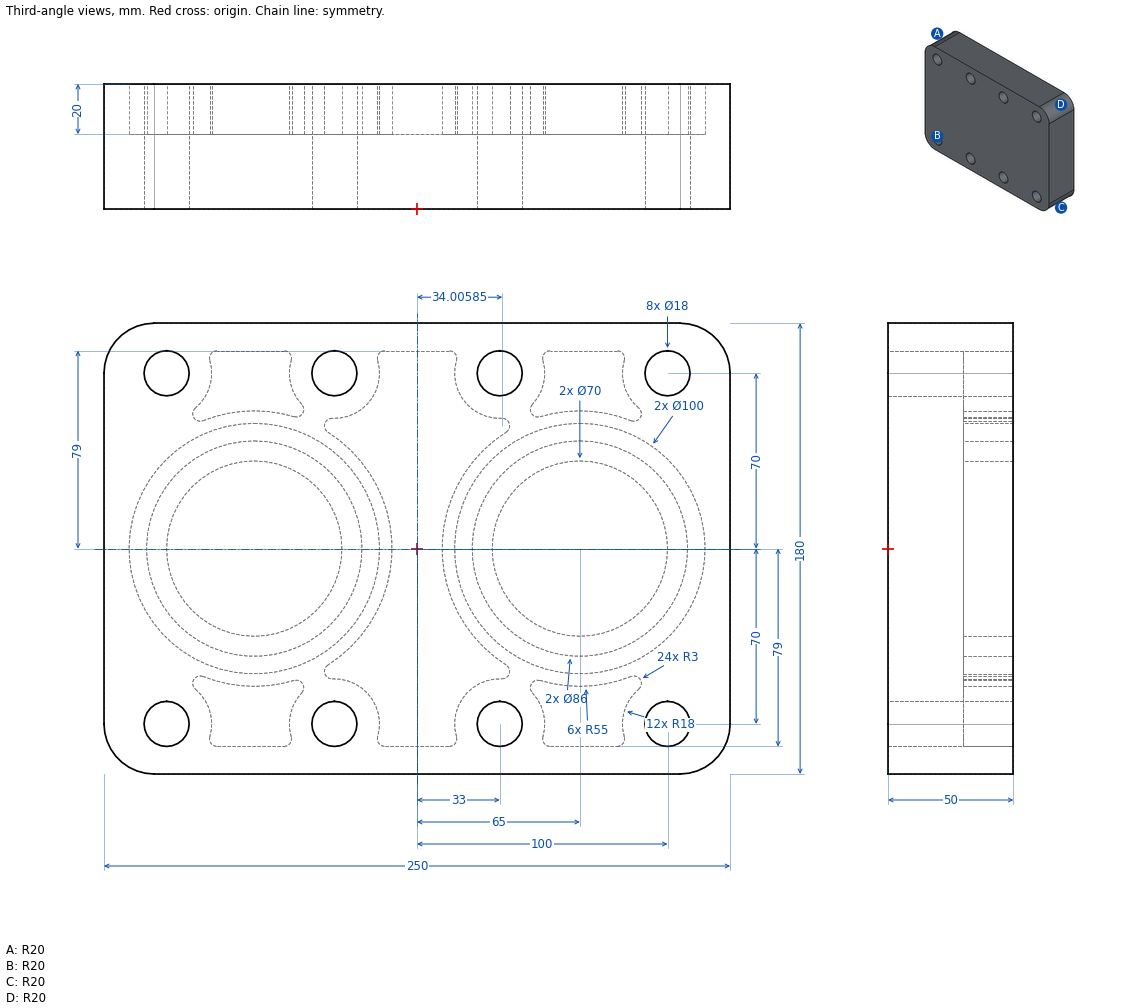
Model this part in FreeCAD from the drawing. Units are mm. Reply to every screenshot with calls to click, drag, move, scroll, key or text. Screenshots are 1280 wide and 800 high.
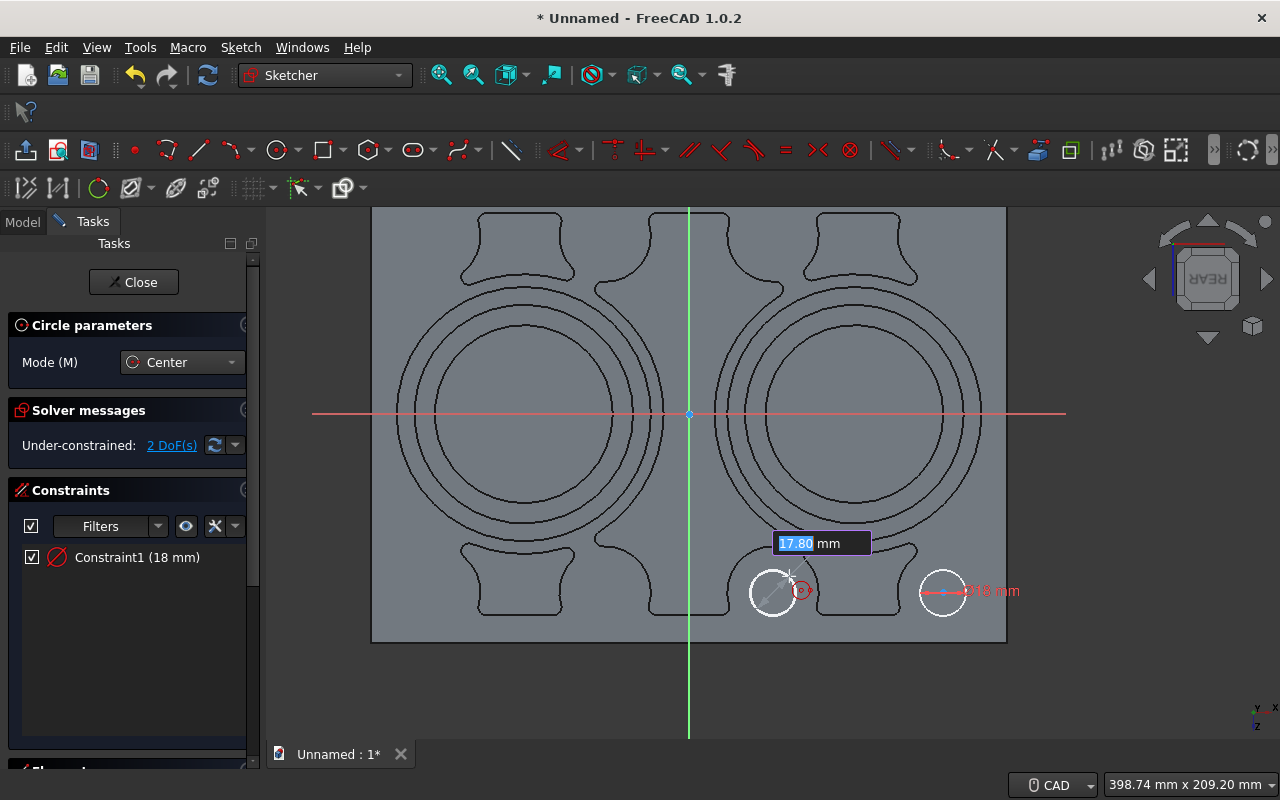
text(18)
key(Return)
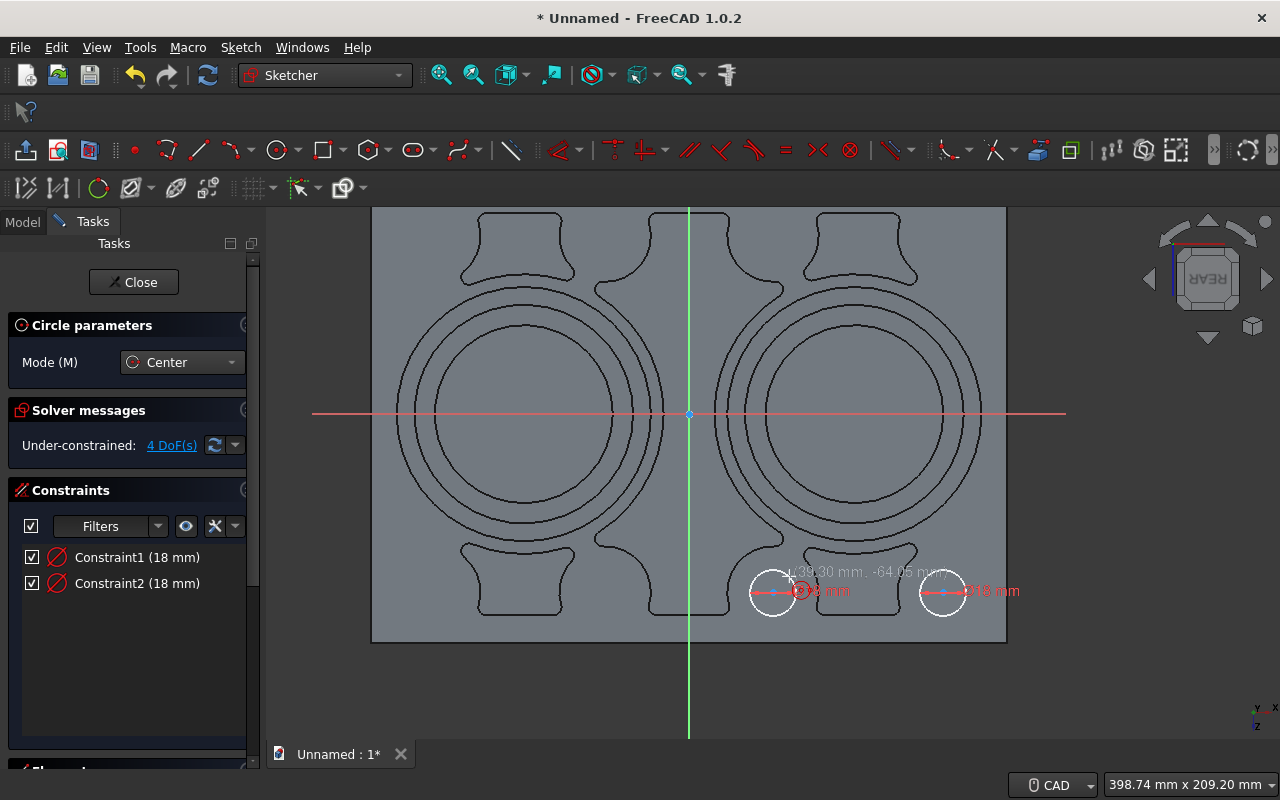
click(605, 592)
move(621, 576)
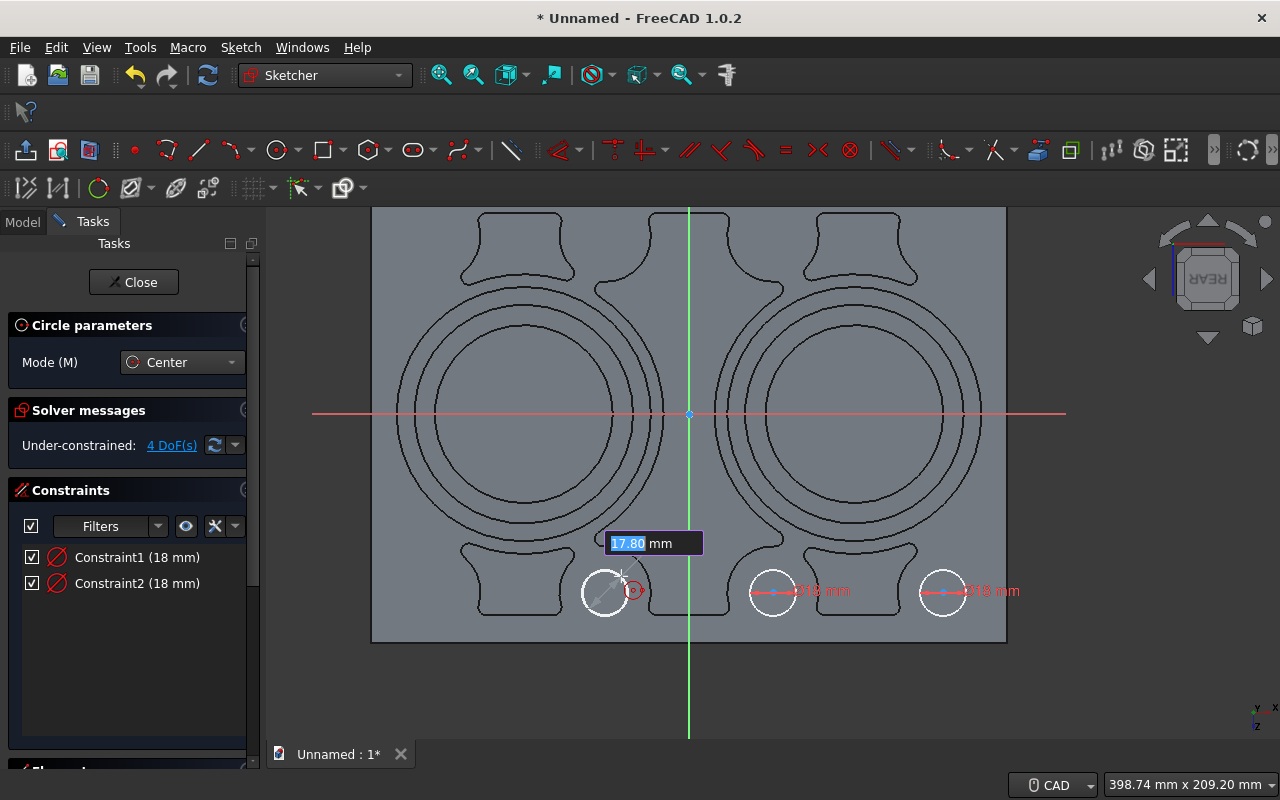
text(18)
key(Return)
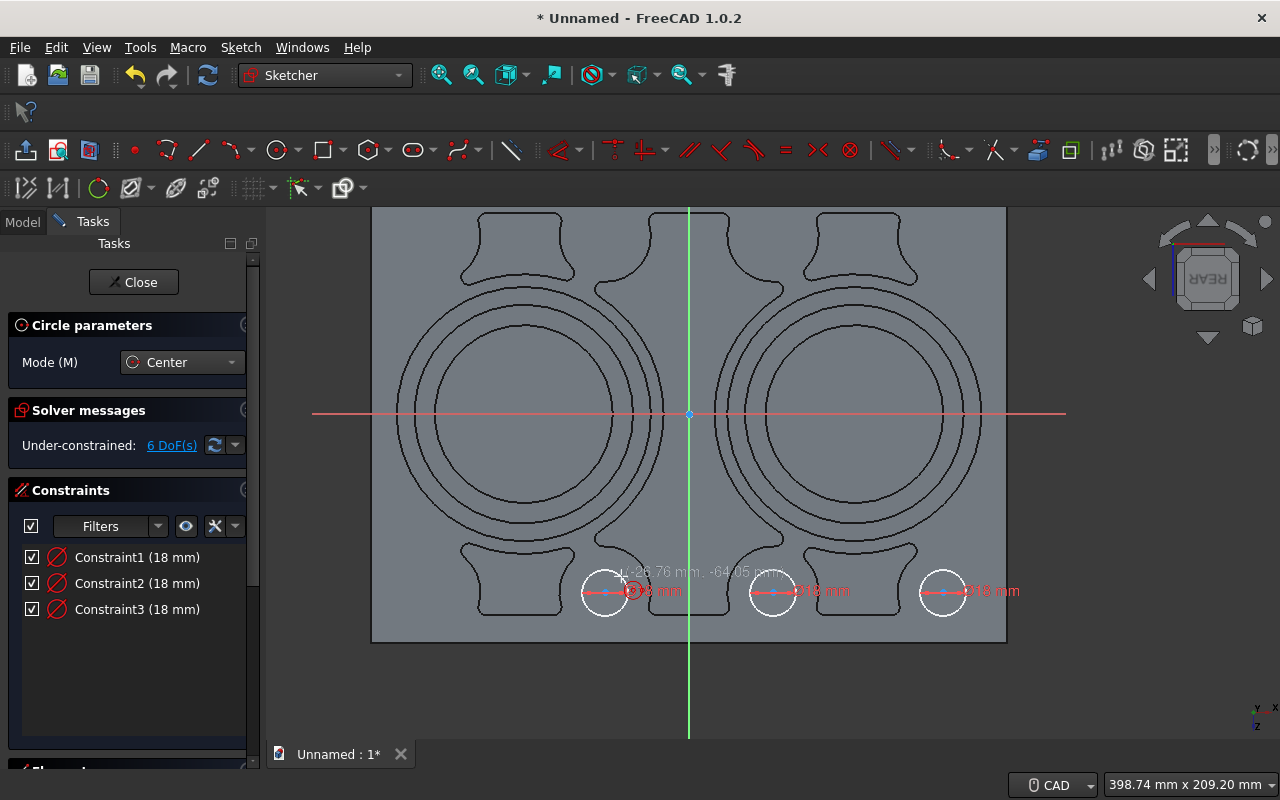
click(435, 592)
move(451, 576)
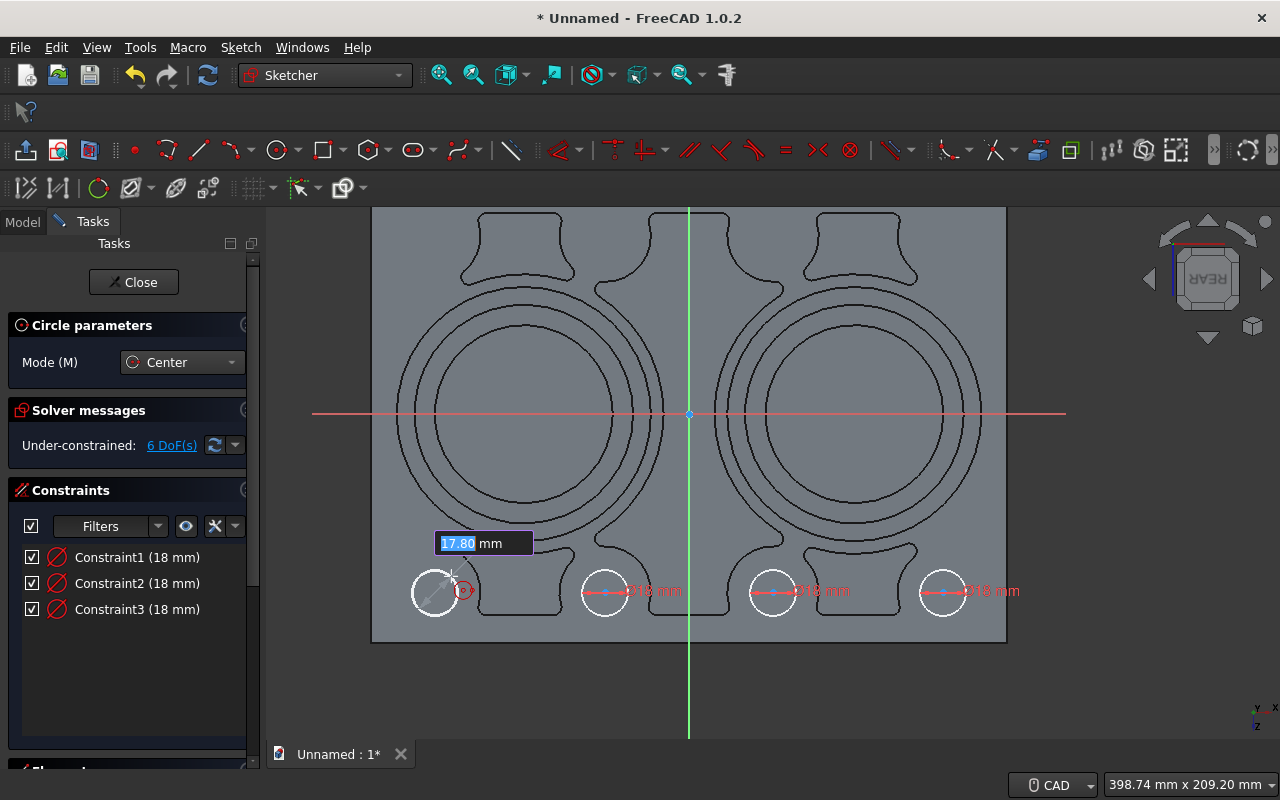
text(18)
key(Return)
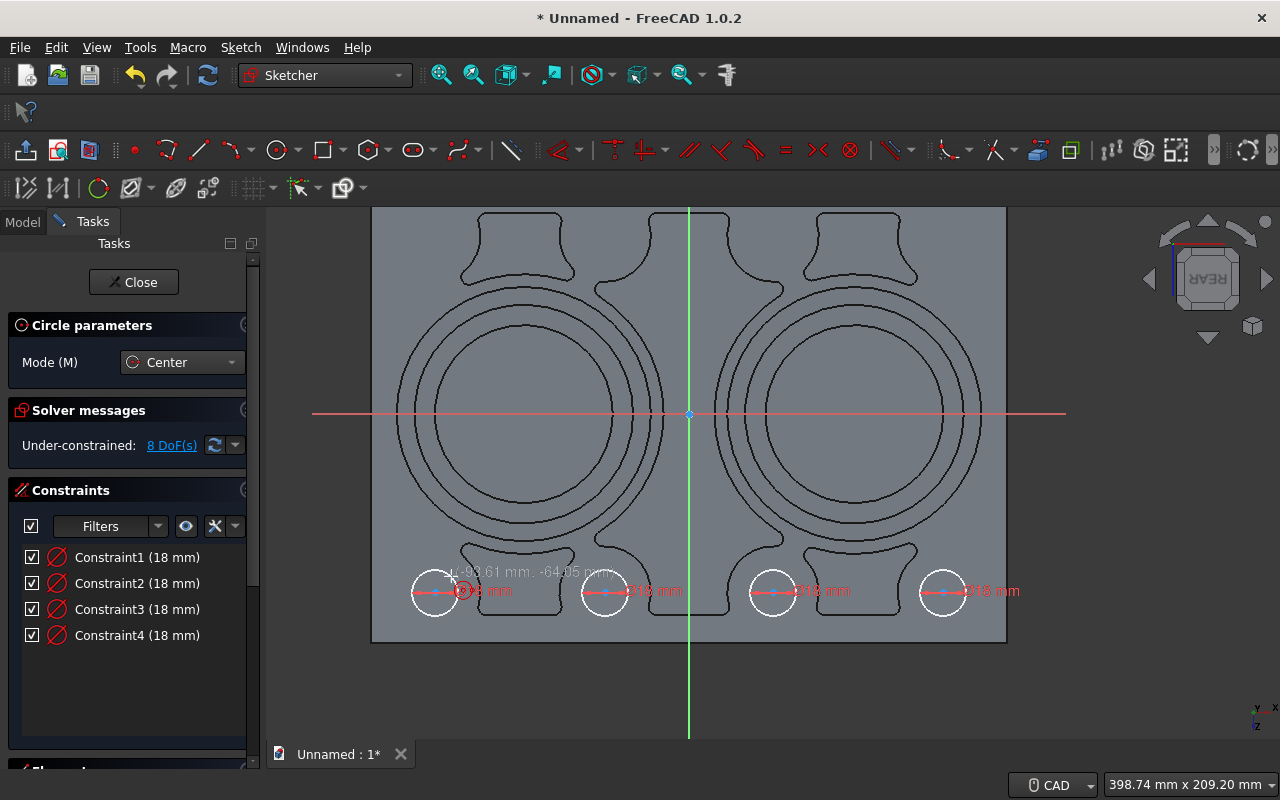
click(435, 236)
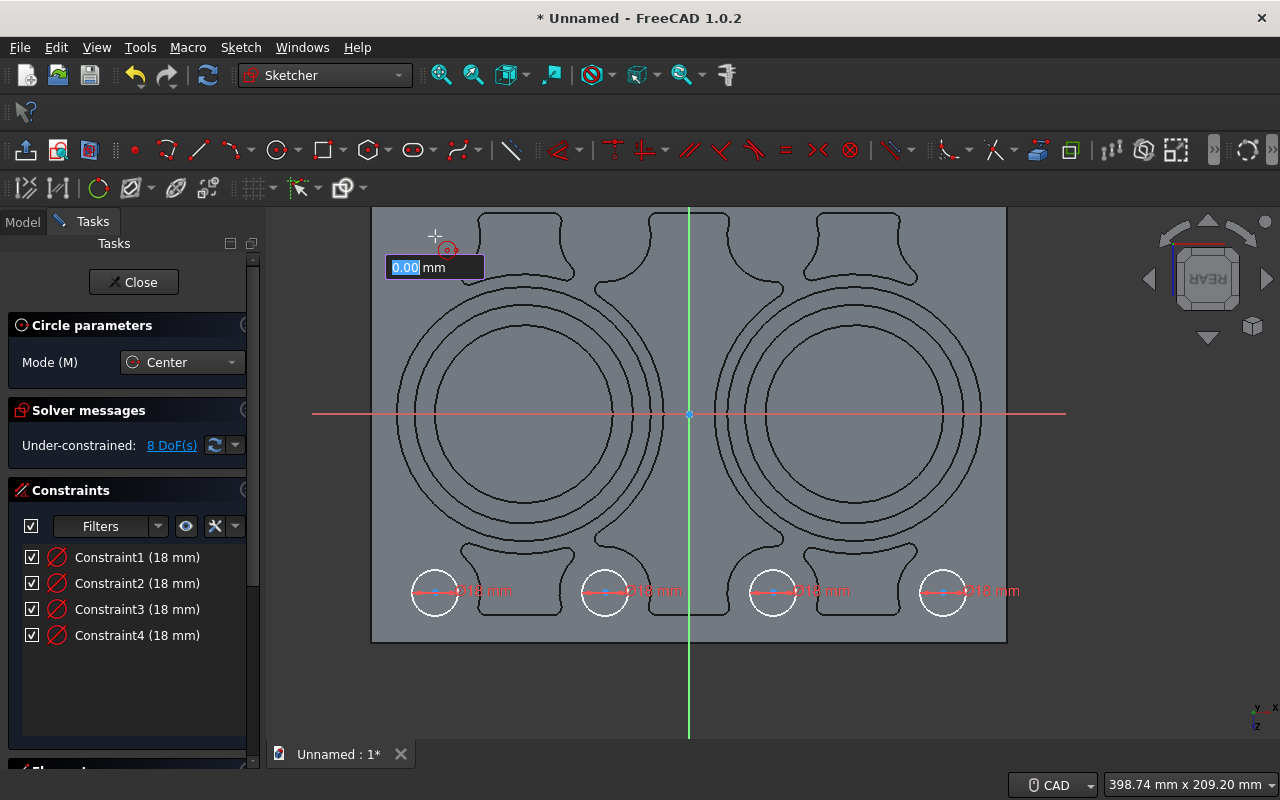
scroll(774, 711, down, 1)
move(510, 309)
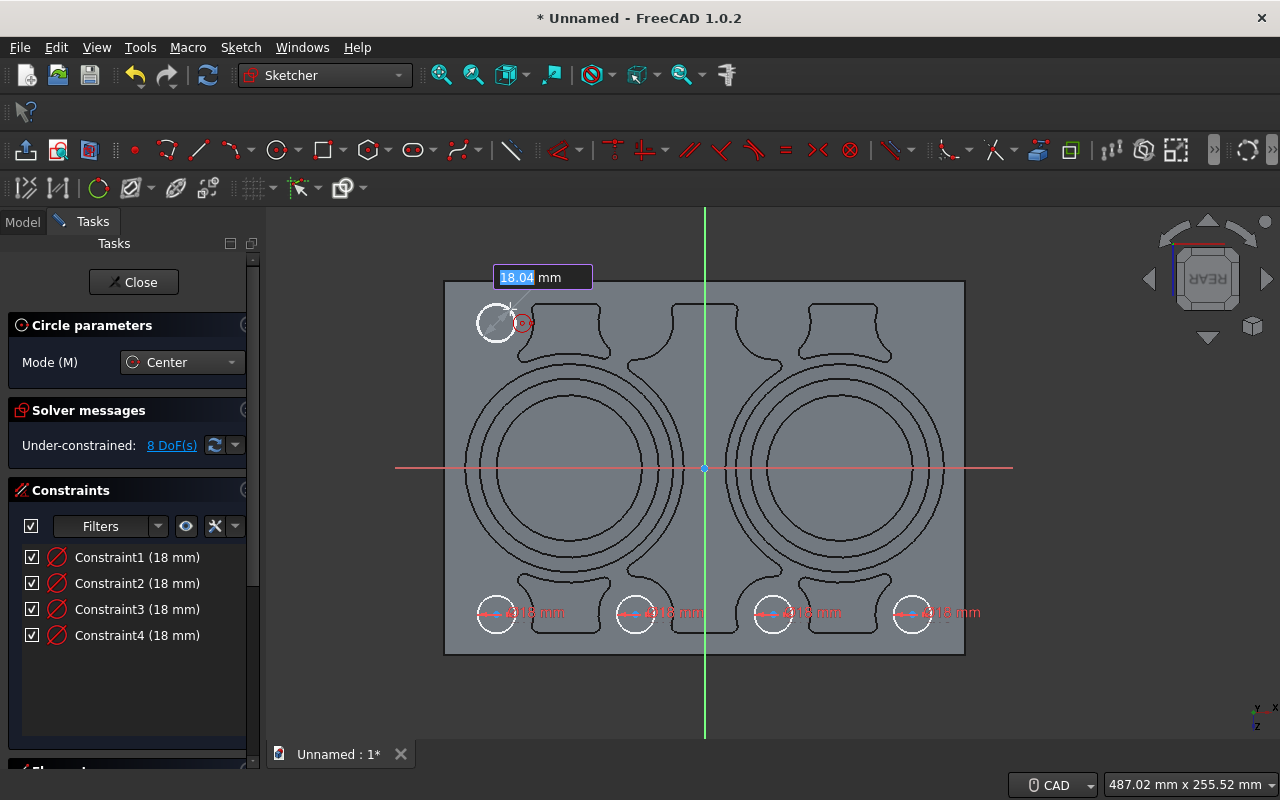
text(18)
key(Return)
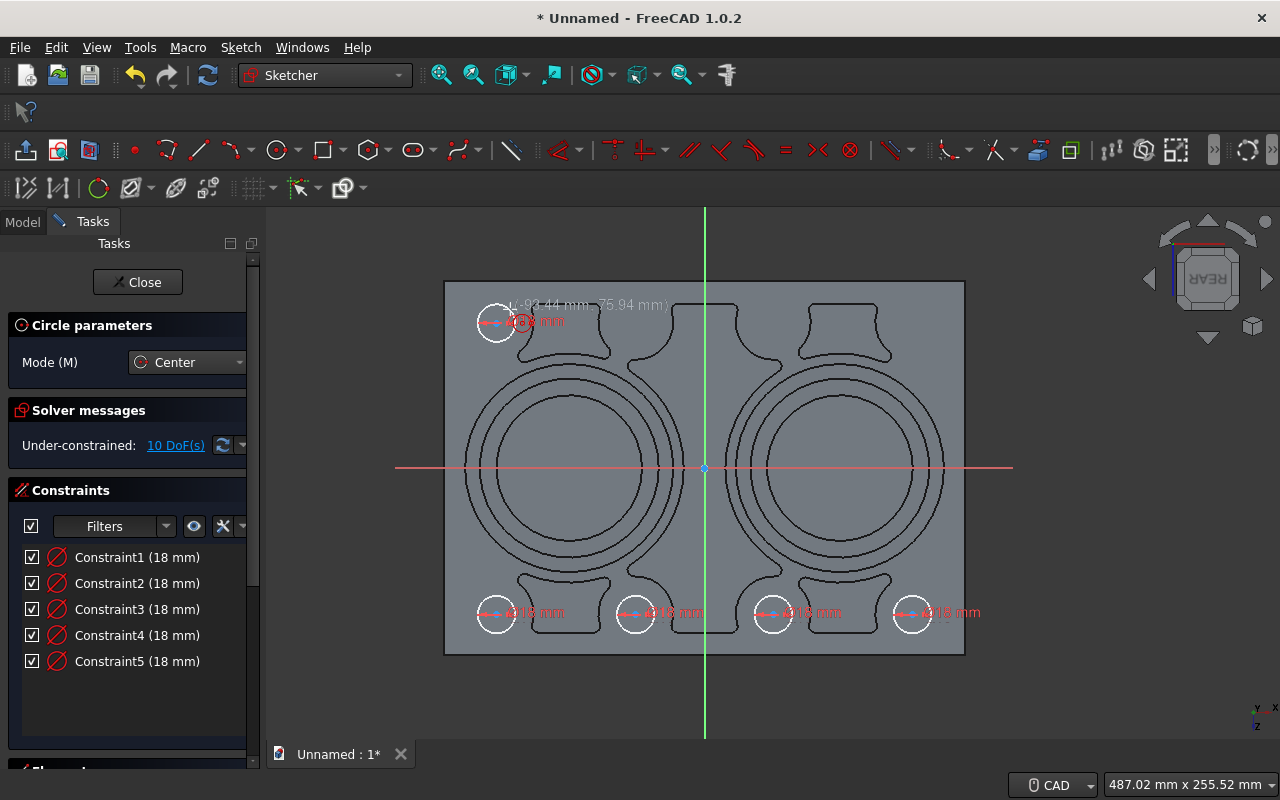
click(636, 322)
move(649, 309)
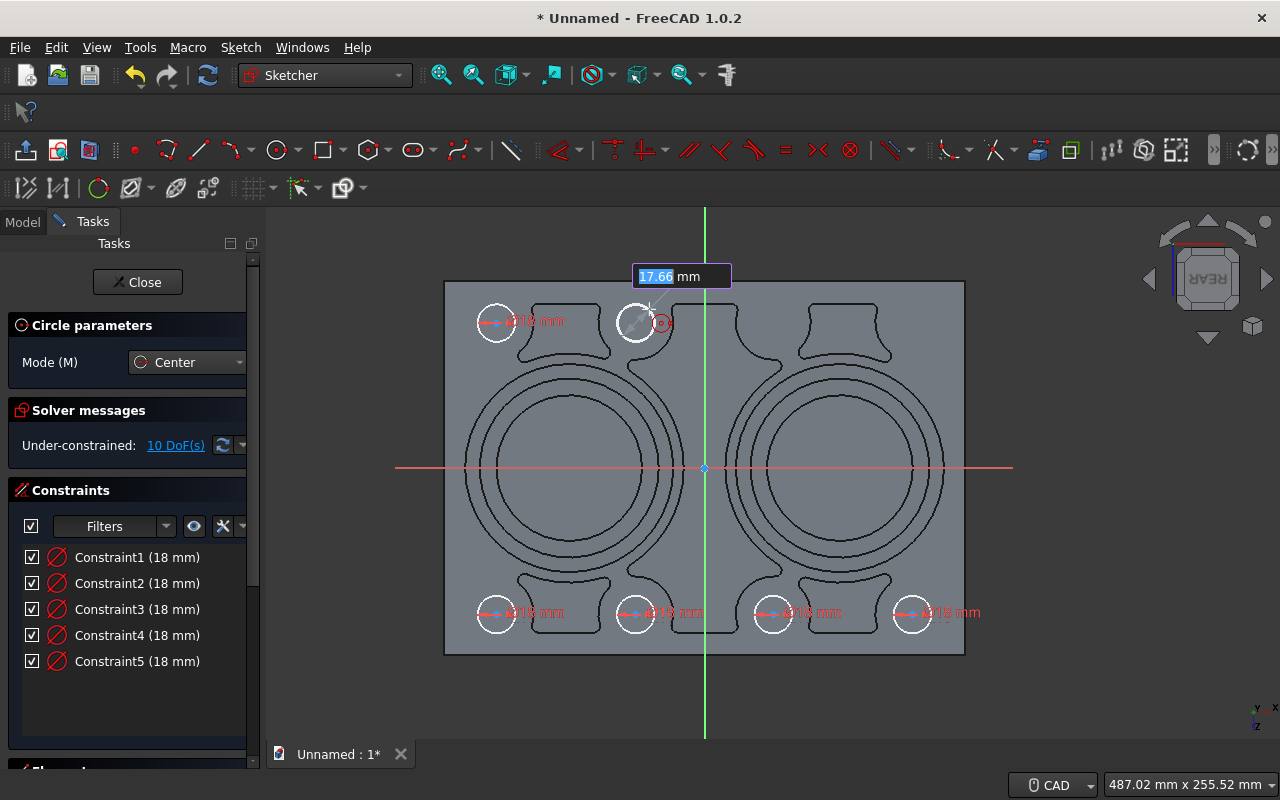
text(18)
key(Return)